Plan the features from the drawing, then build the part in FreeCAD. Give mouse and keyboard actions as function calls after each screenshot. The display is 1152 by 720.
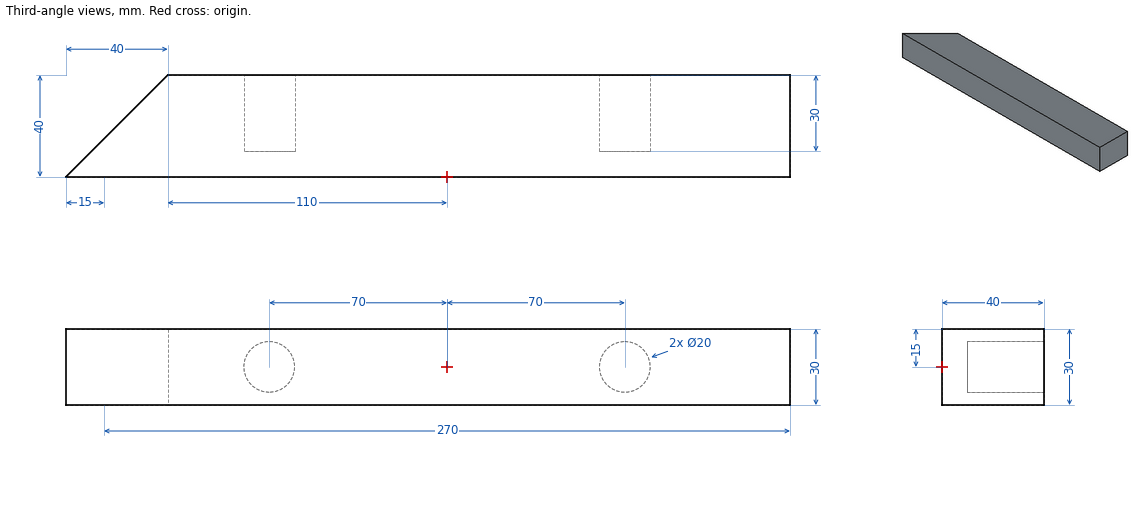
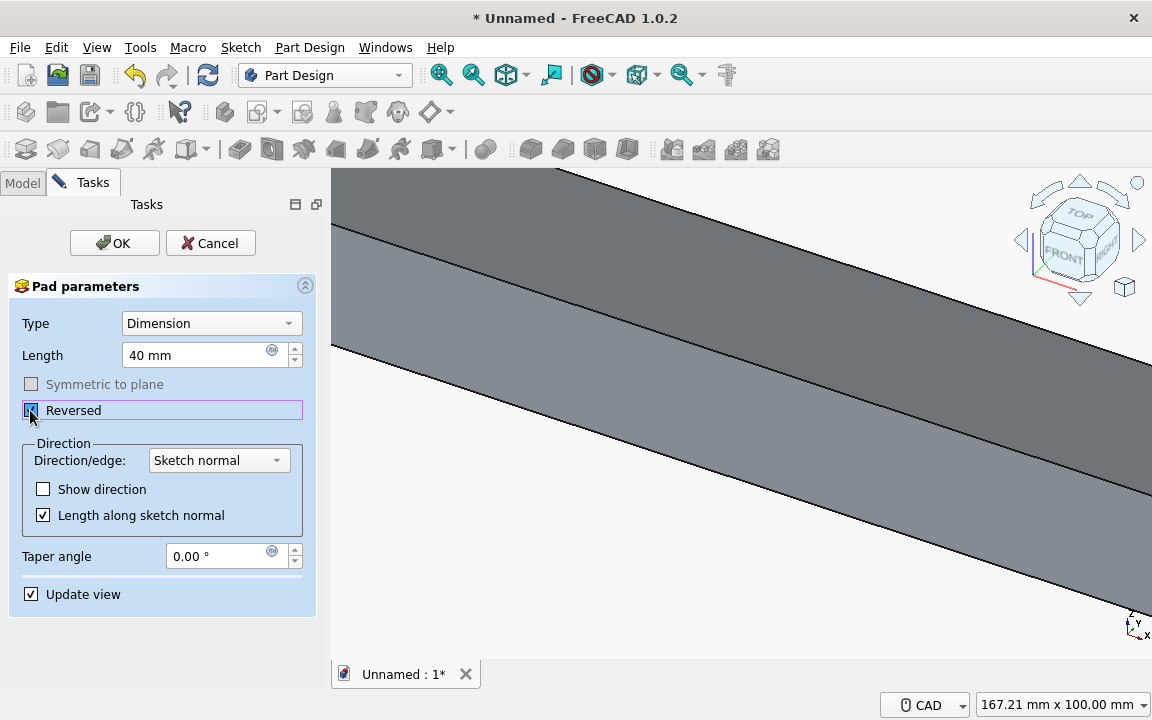
click(115, 243)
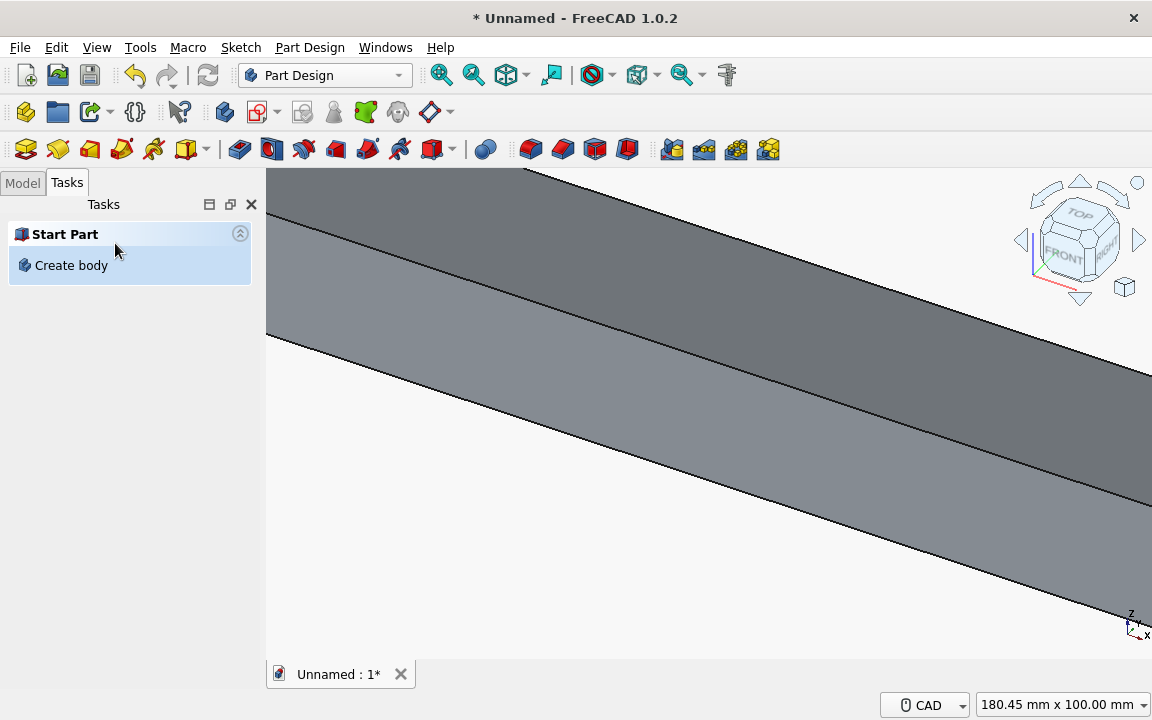
key(v)
key(f)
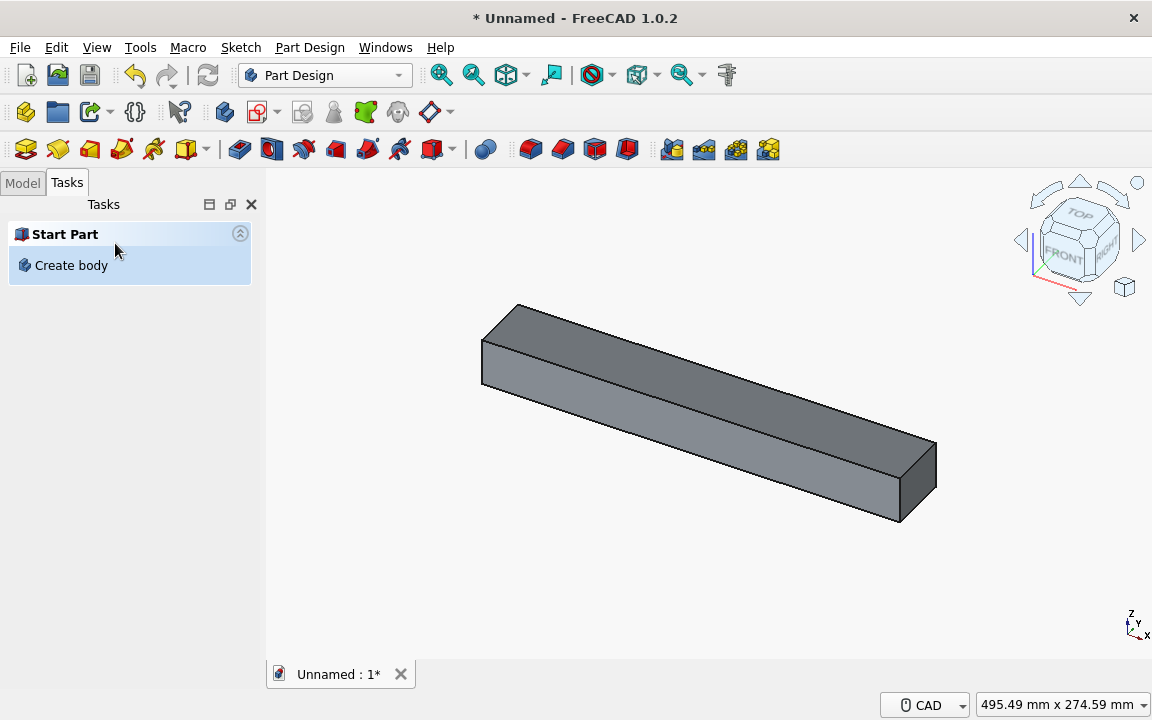
key(4)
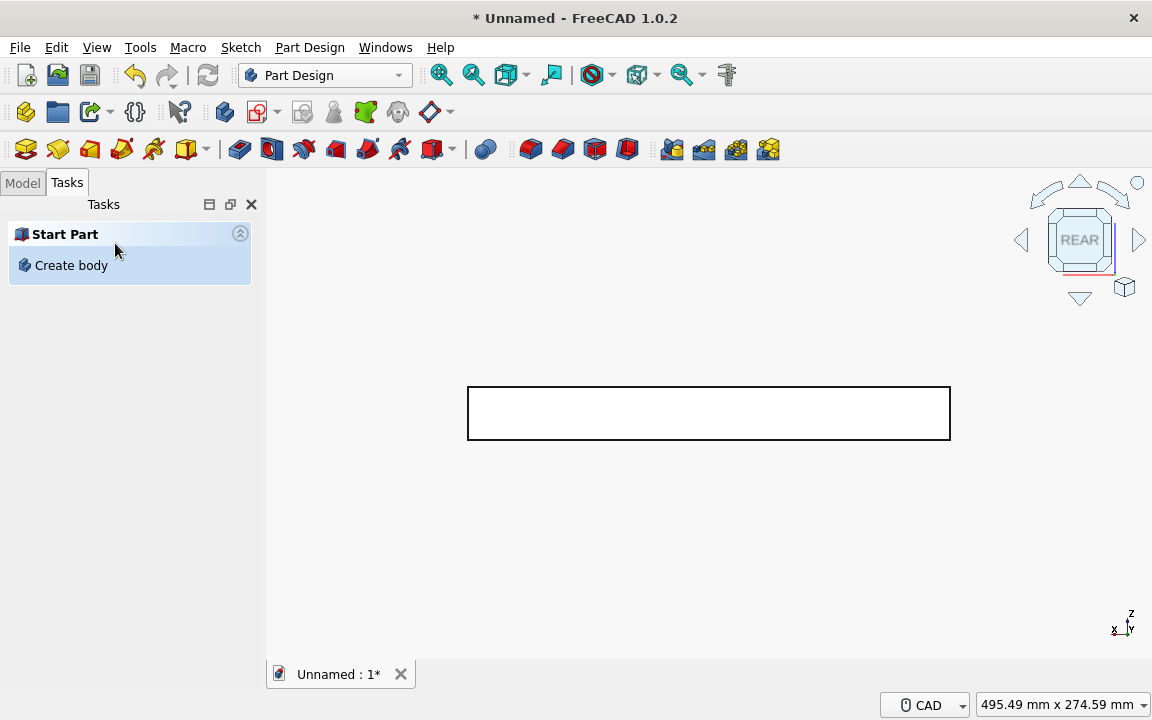
click(502, 413)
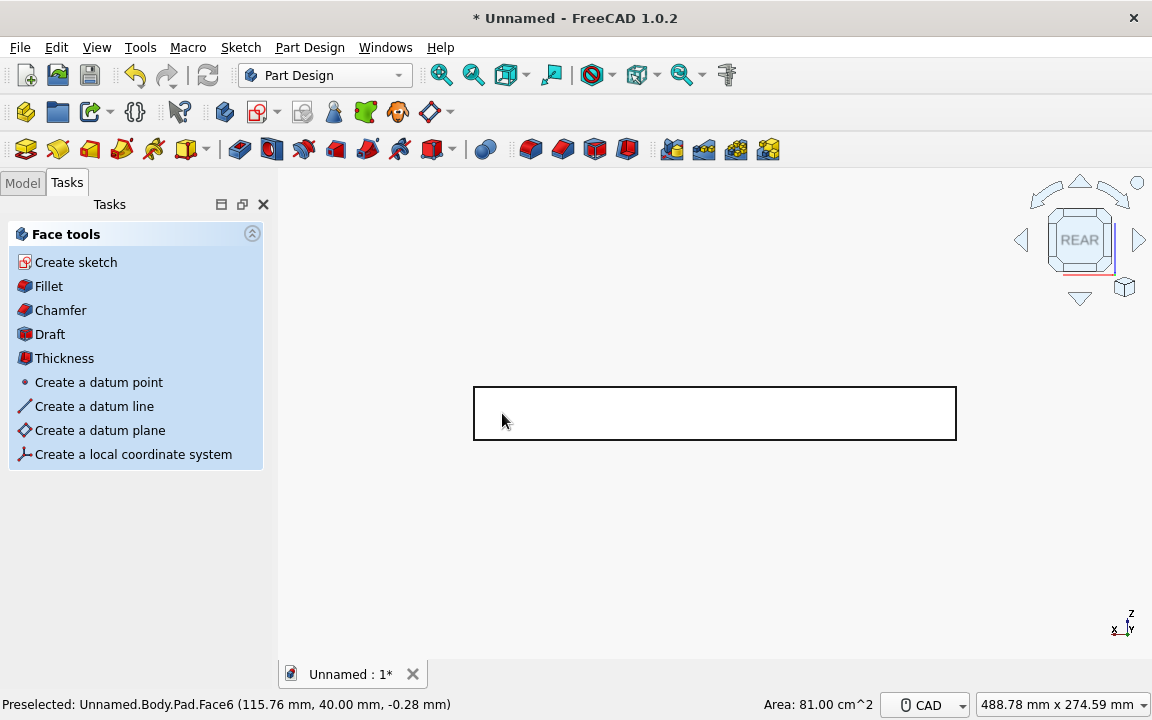
click(258, 112)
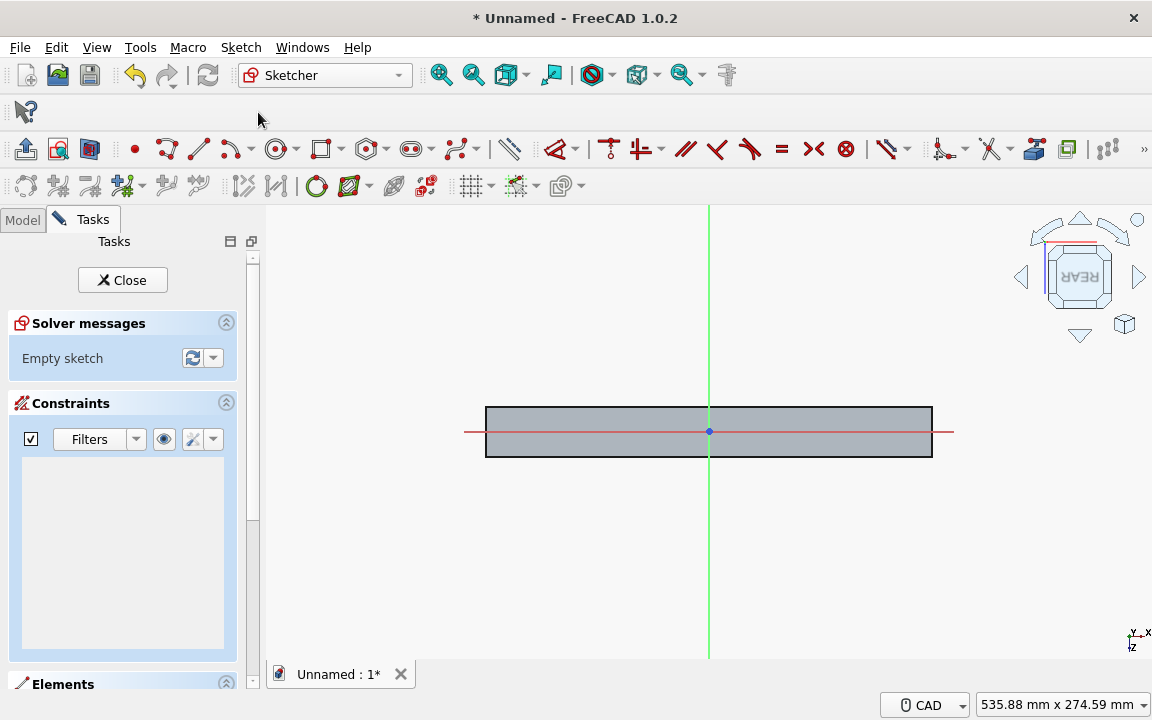
scroll(792, 432, up, 3)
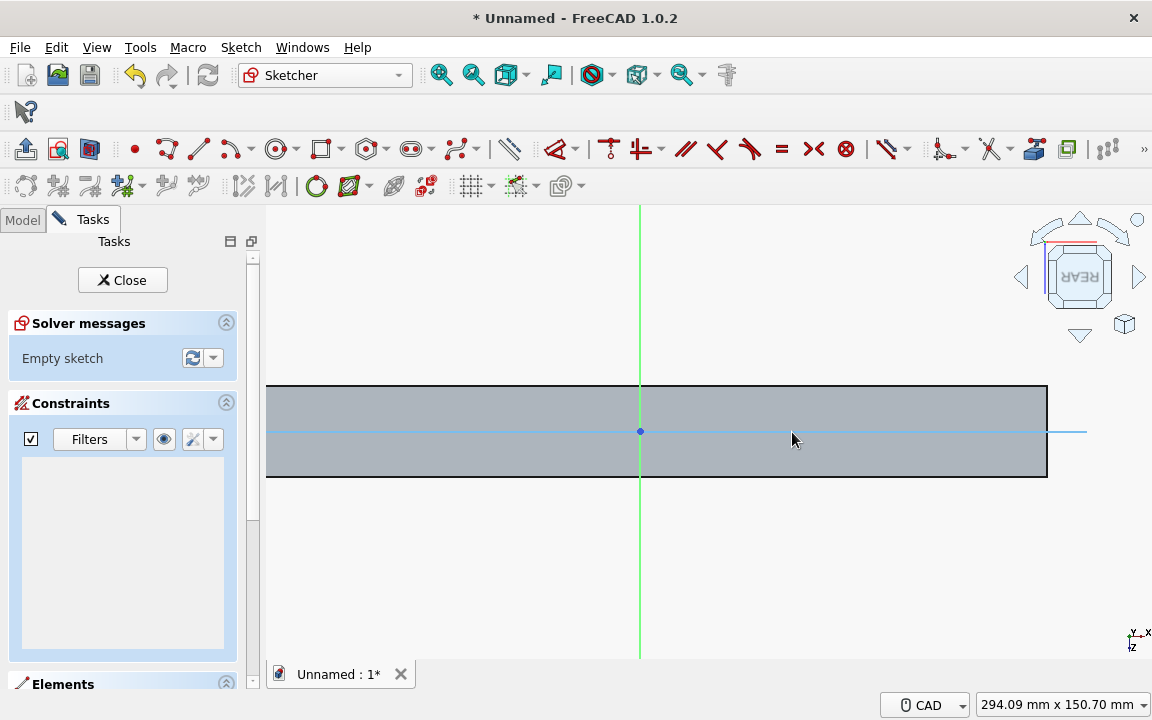
key(g)
key(c)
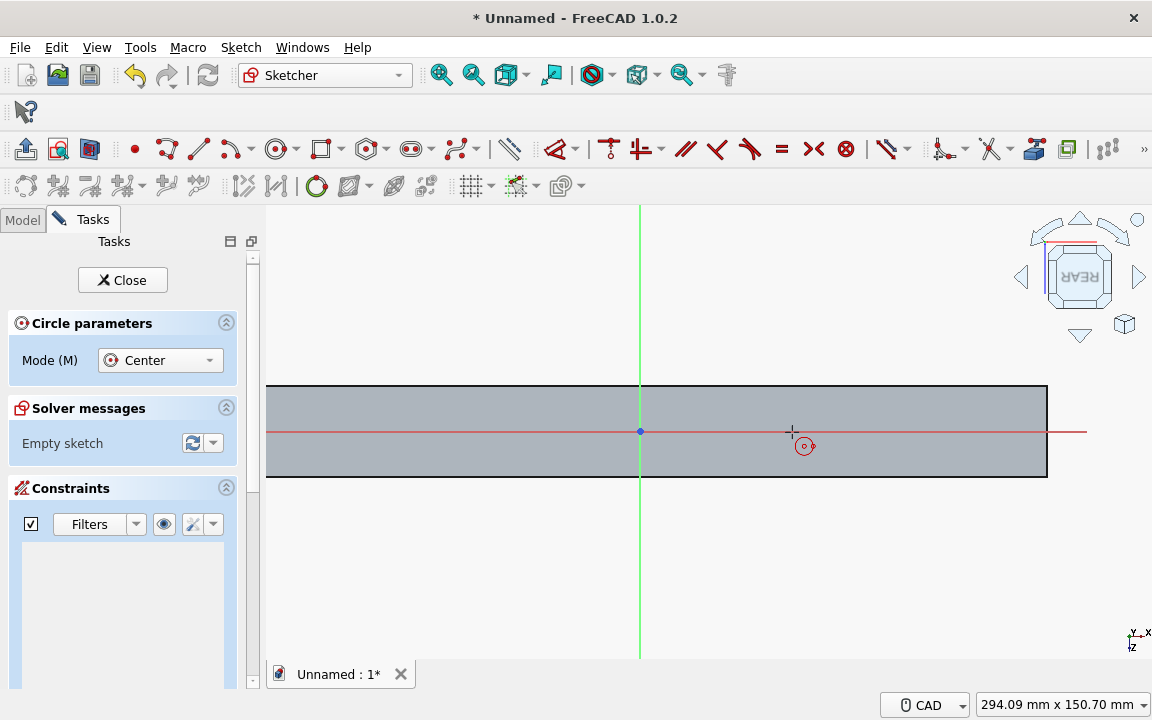
click(851, 432)
move(872, 410)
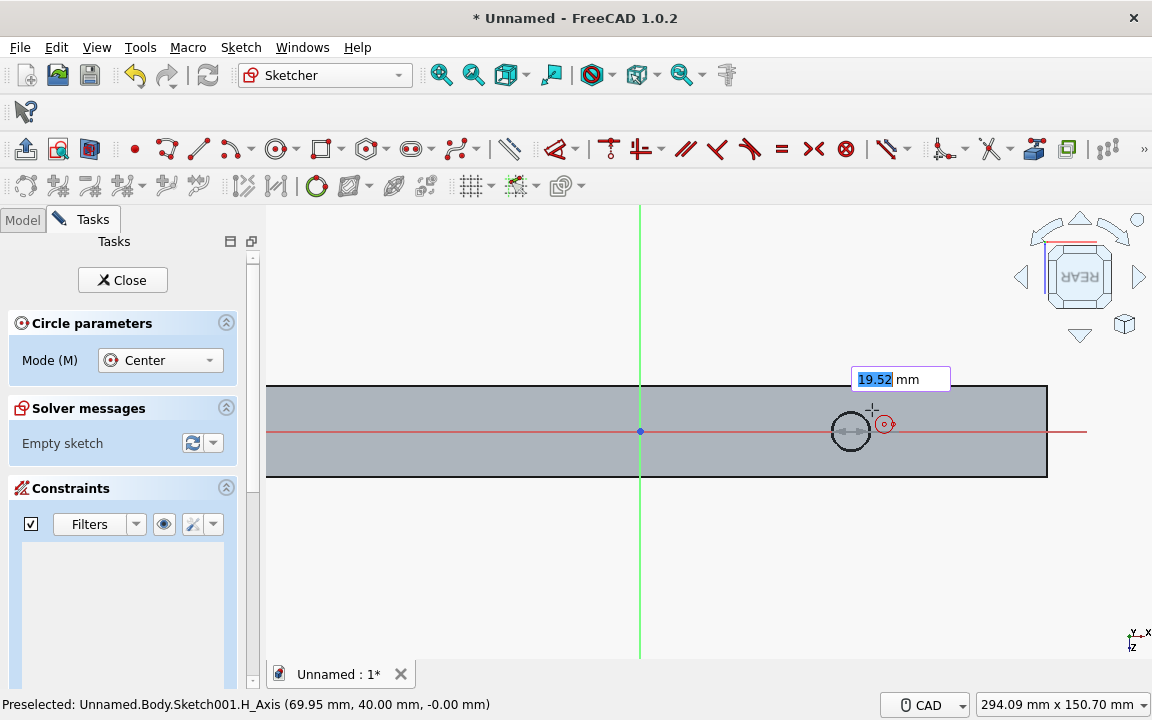
text(20)
key(Return)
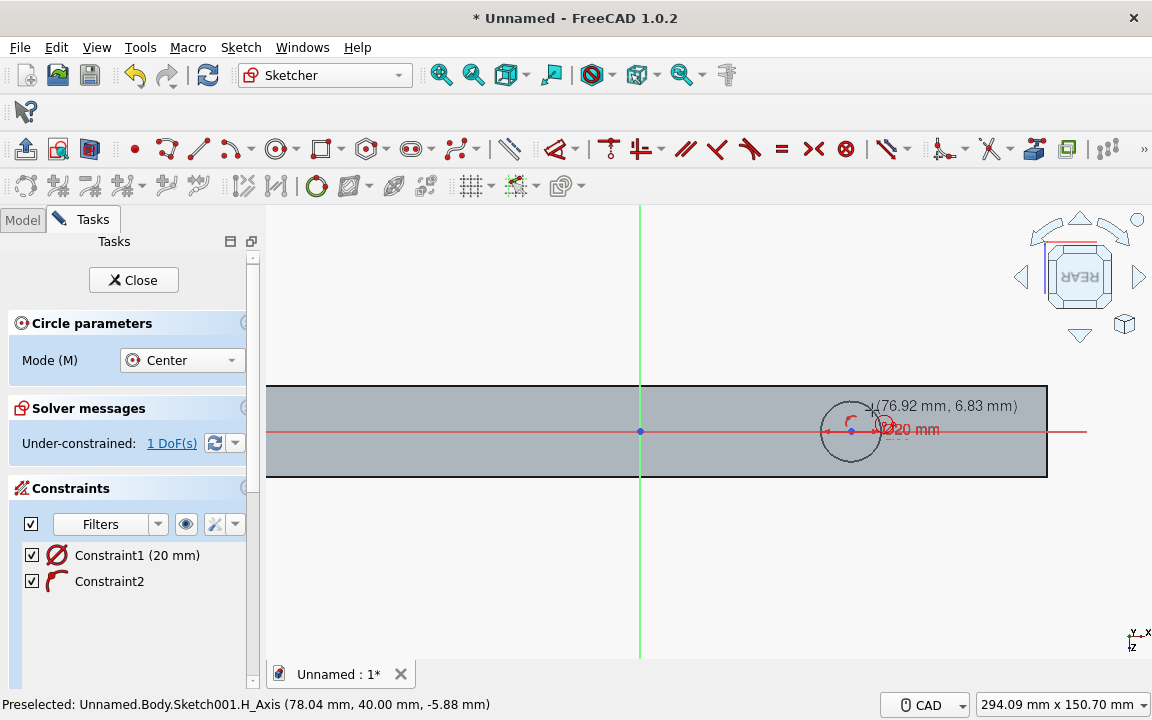
click(429, 432)
move(451, 410)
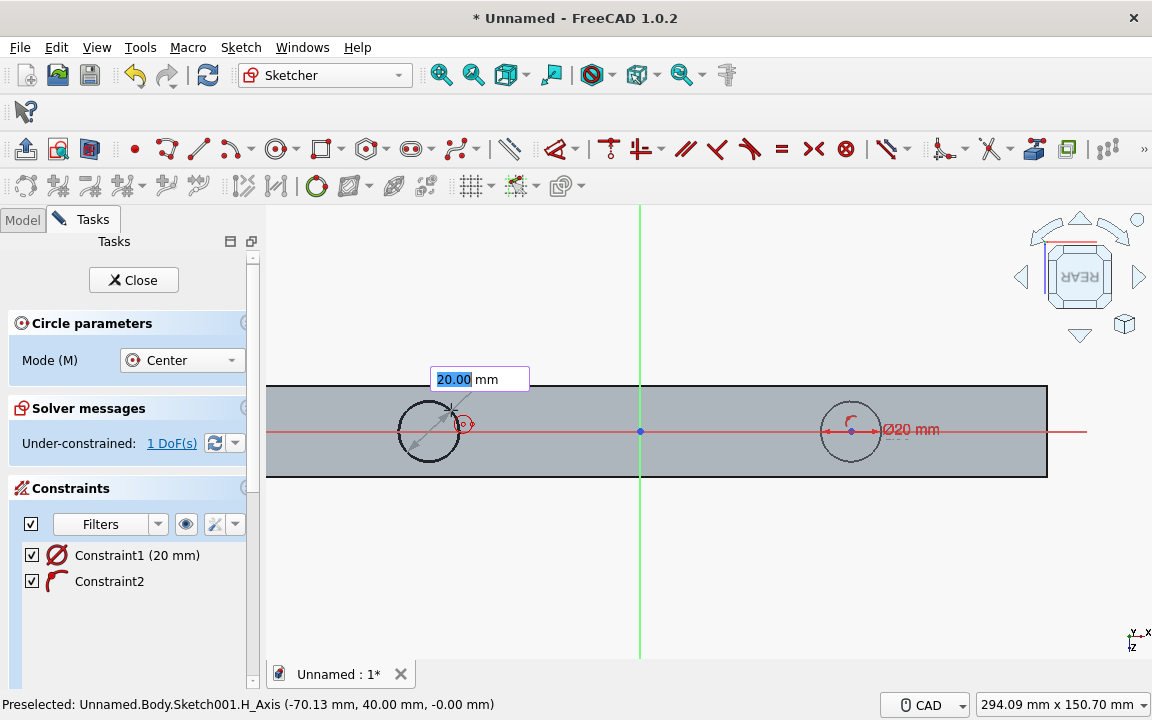
text(20)
key(Return)
key(Escape)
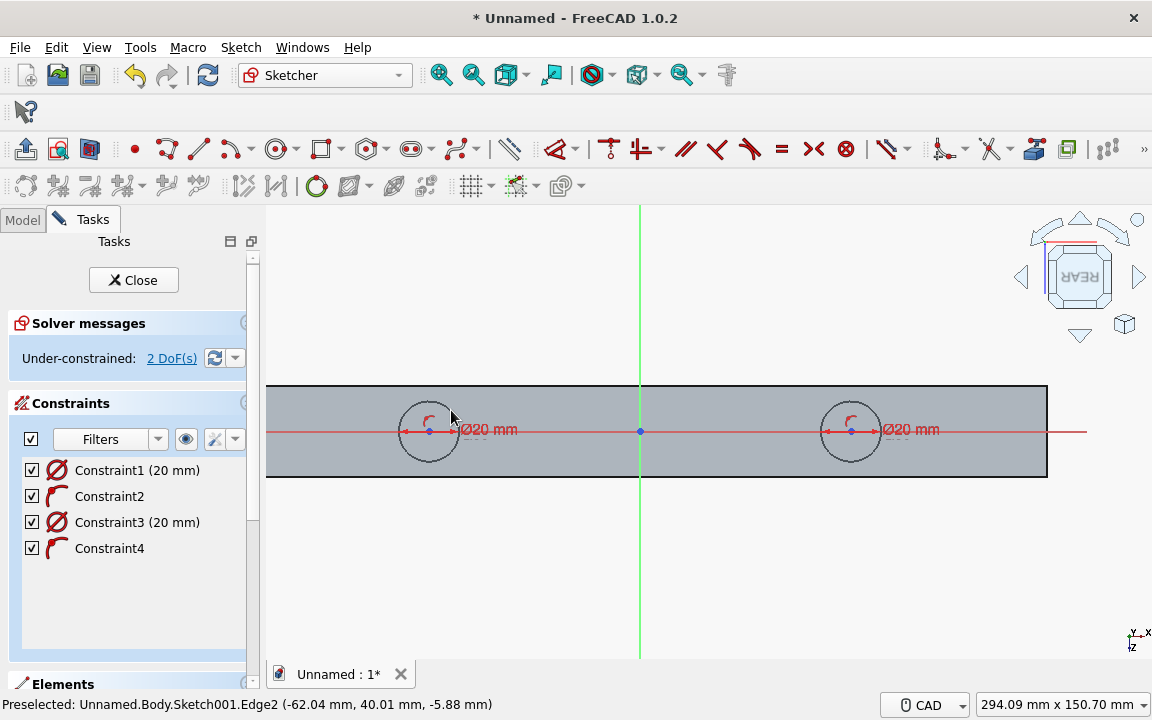
click(556, 150)